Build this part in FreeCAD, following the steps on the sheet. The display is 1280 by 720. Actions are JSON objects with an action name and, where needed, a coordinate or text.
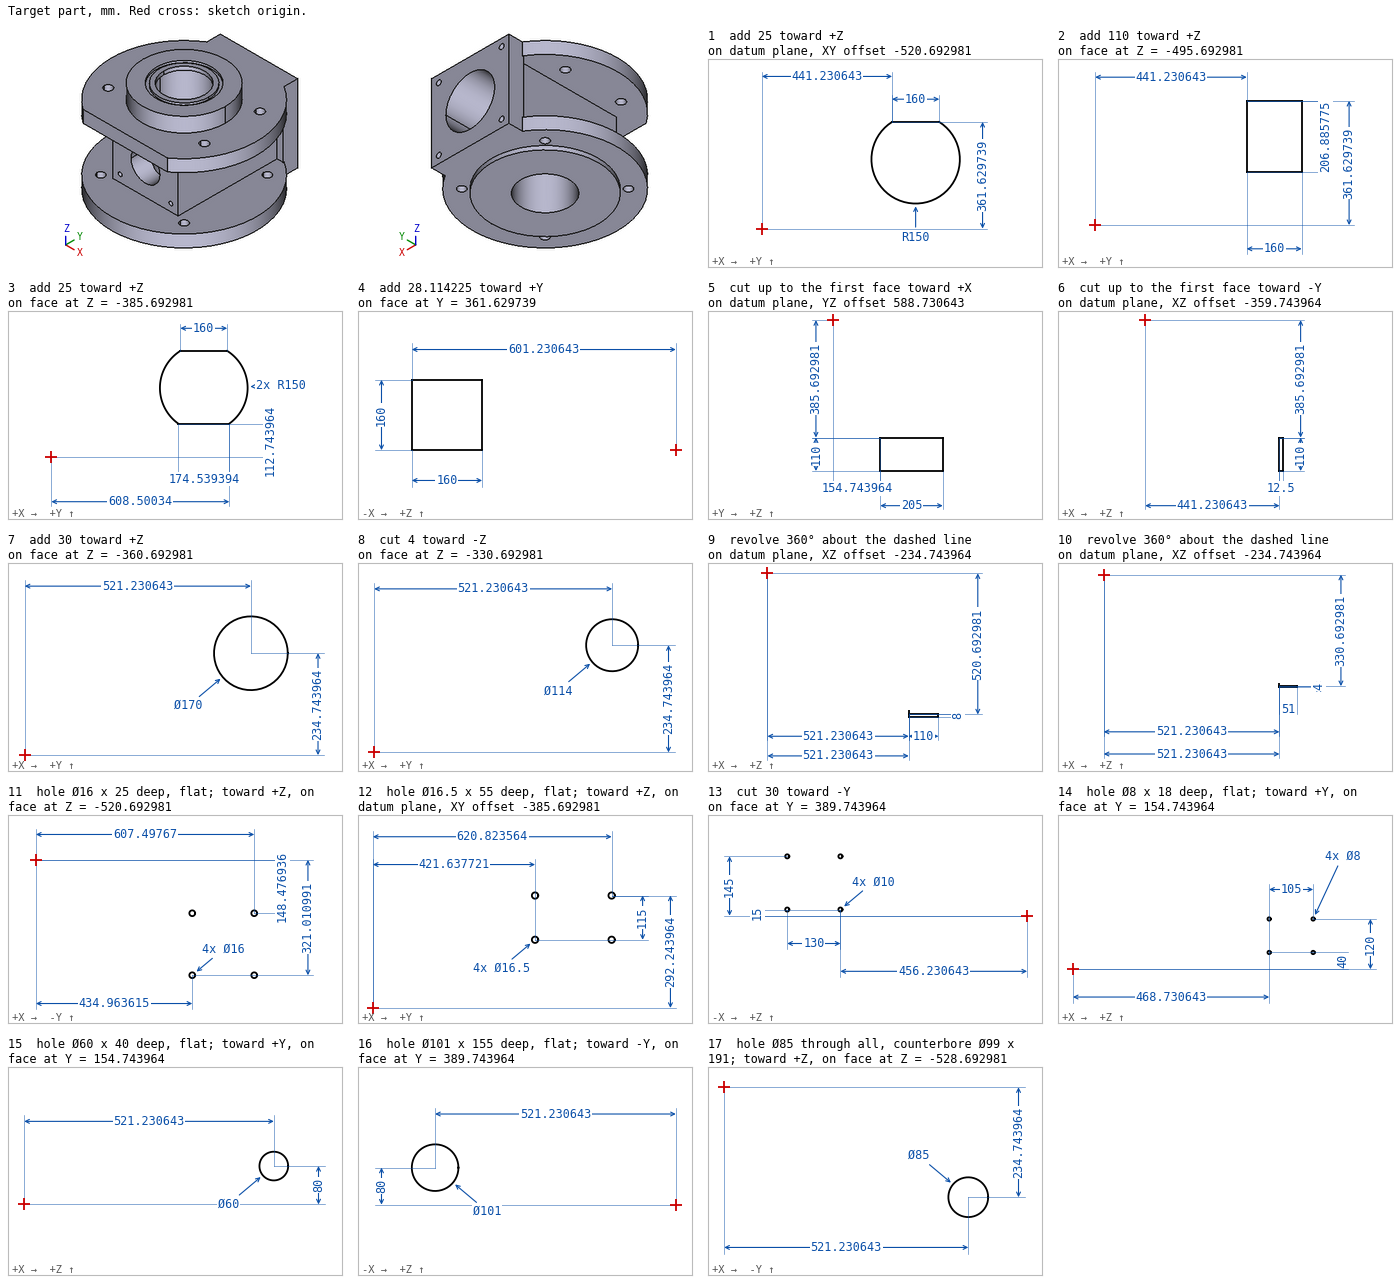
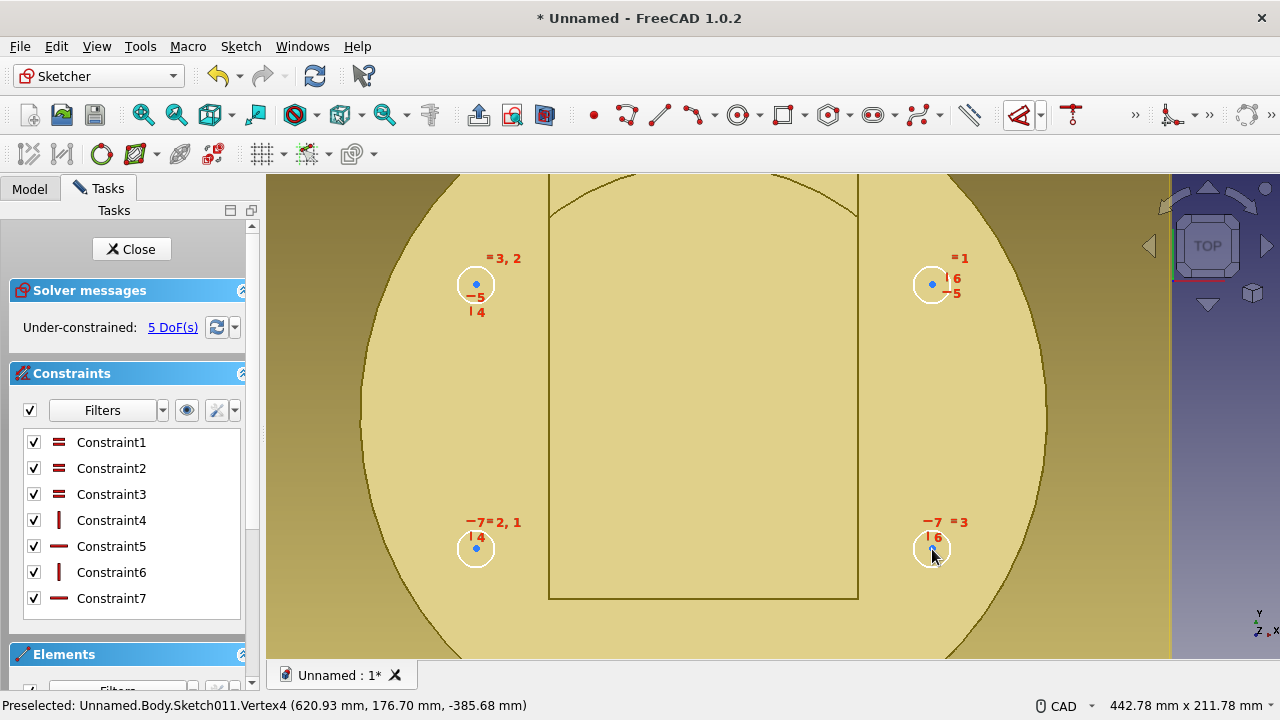
{"action": "left_click", "coordinate": [919, 272]}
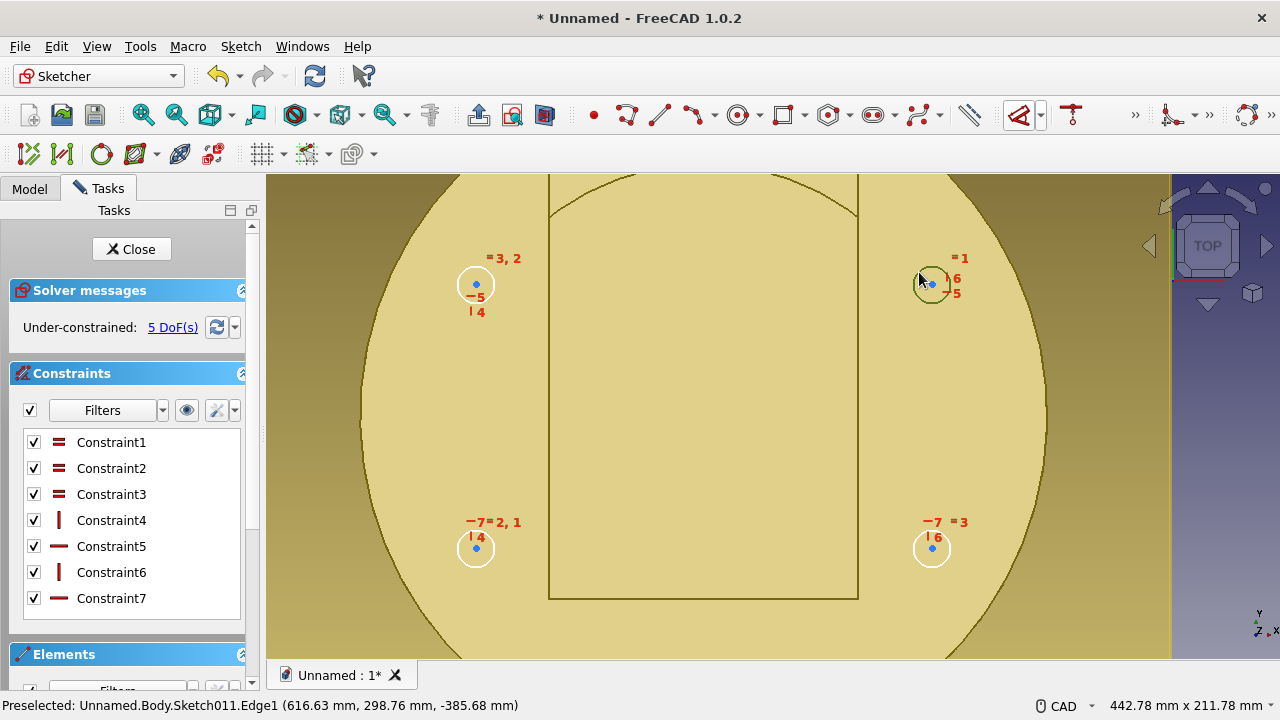
{"action": "left_click", "coordinate": [1040, 116]}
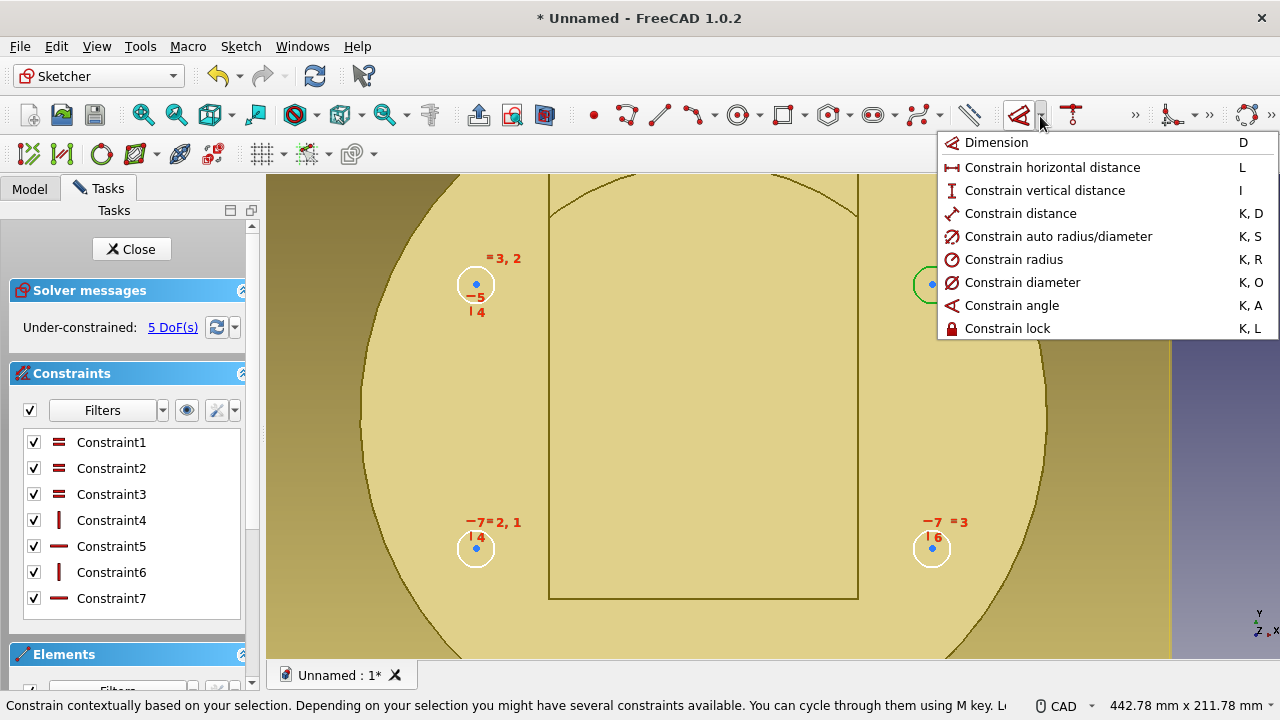
{"action": "left_click", "coordinate": [1108, 282]}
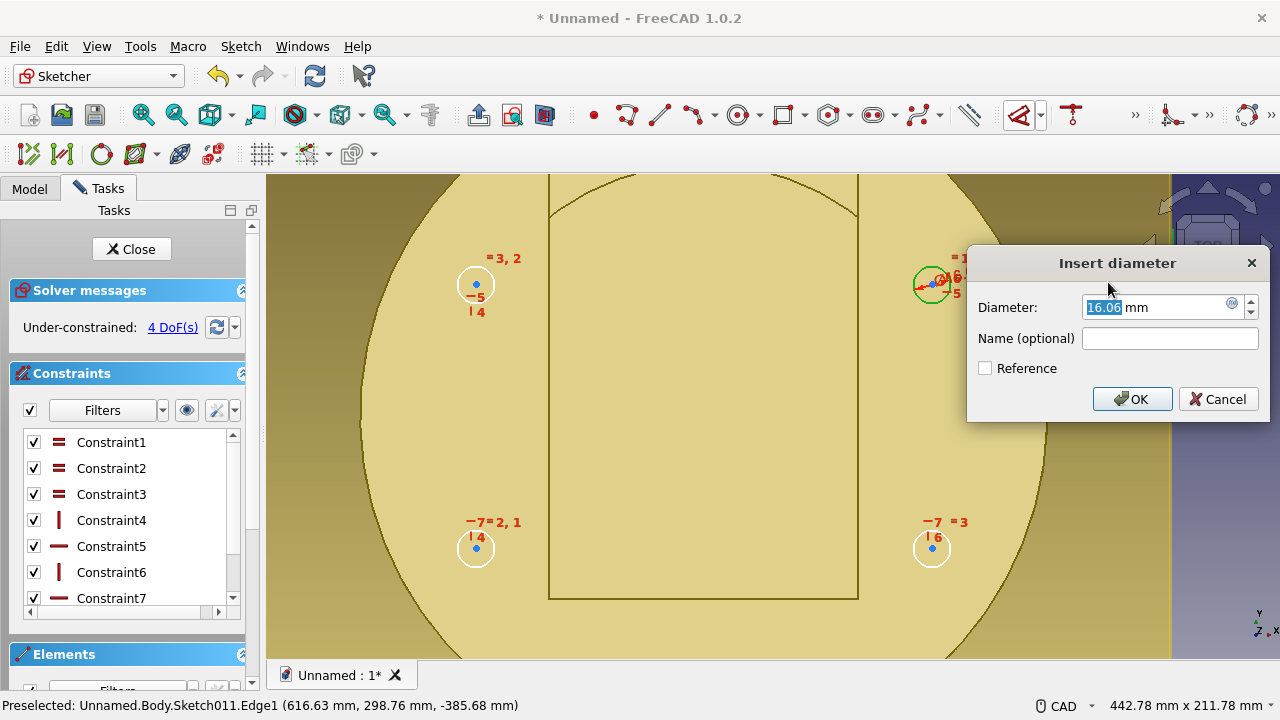
{"action": "type", "text": "16.5"}
{"action": "key", "text": "Return"}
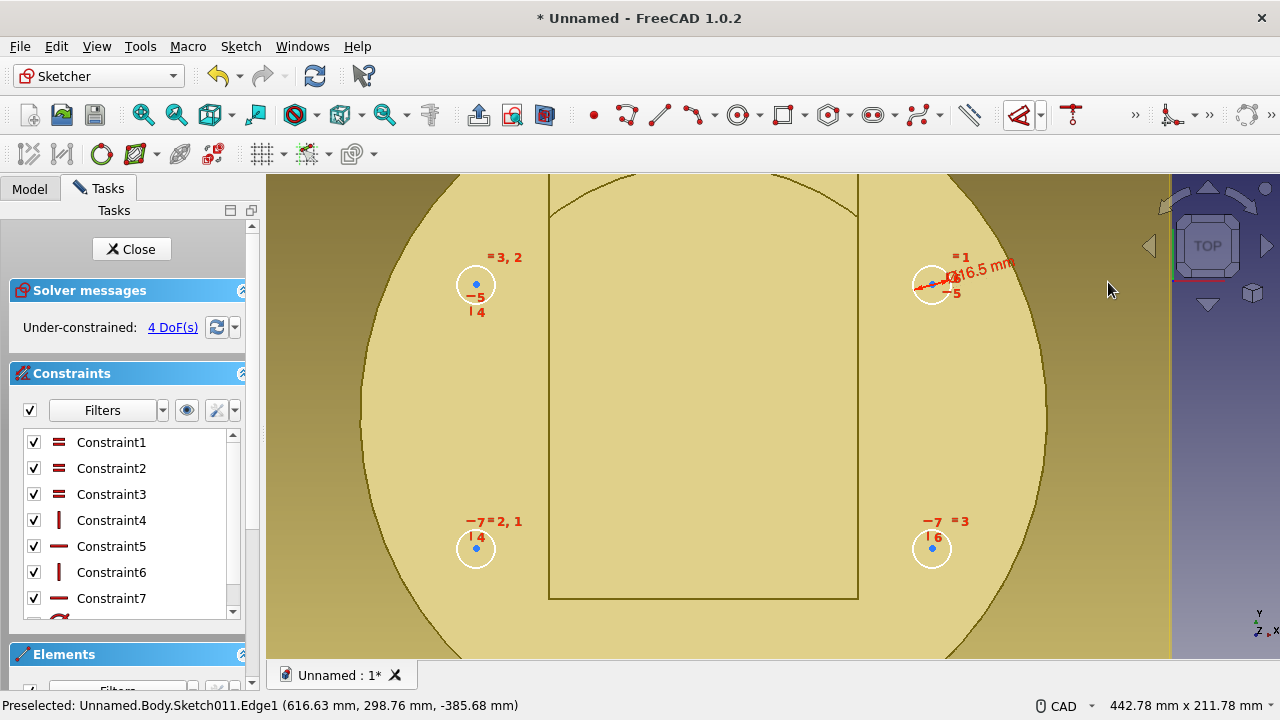
{"action": "left_click", "coordinate": [932, 285]}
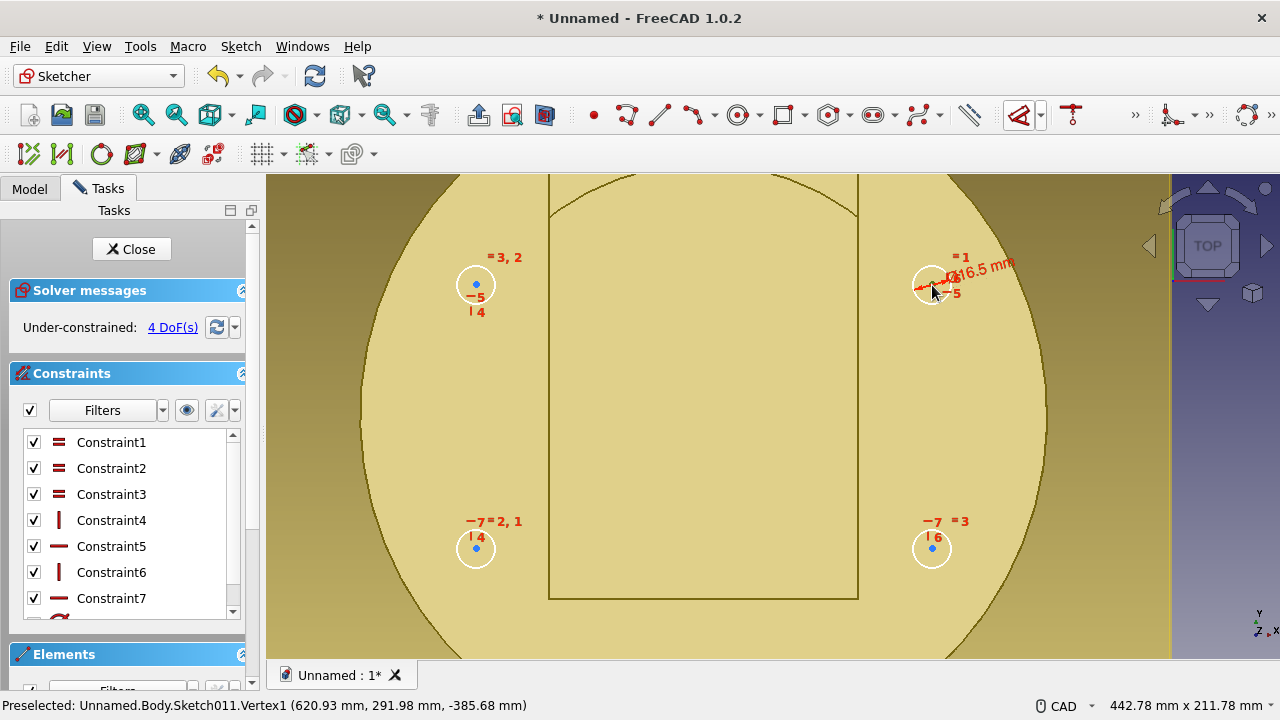
{"action": "left_click", "coordinate": [476, 549]}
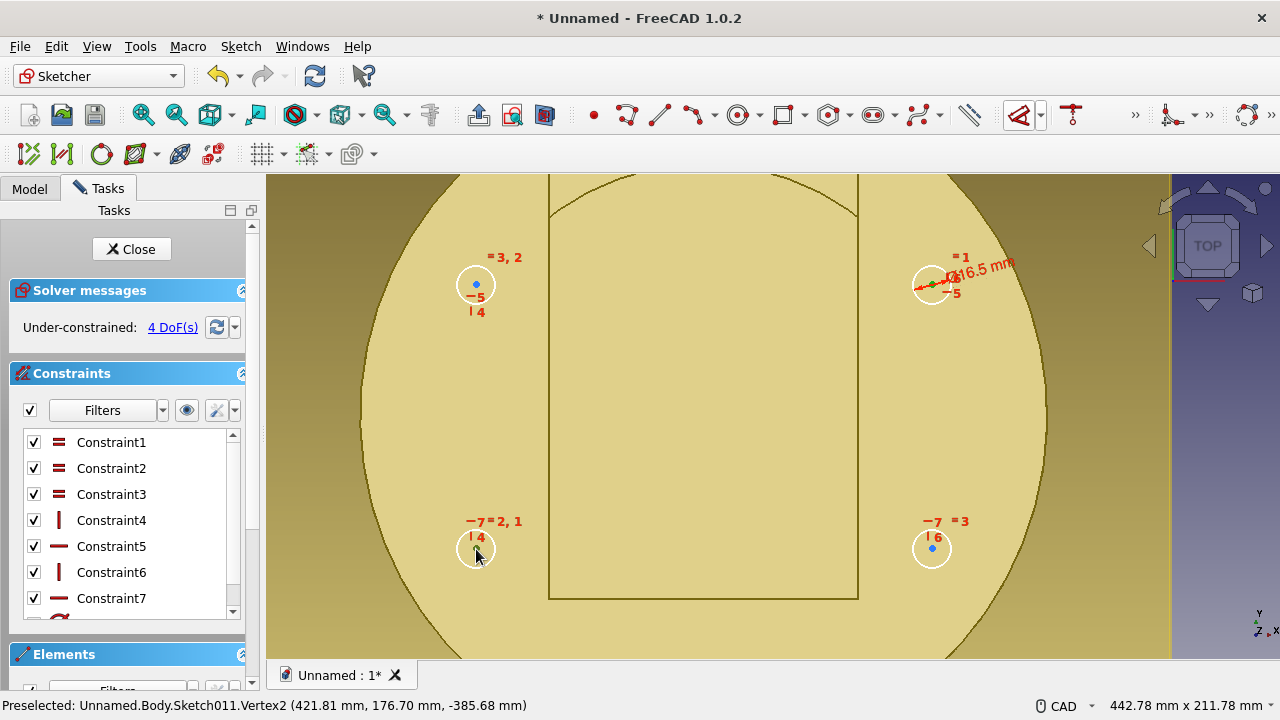
{"action": "left_click", "coordinate": [1040, 116]}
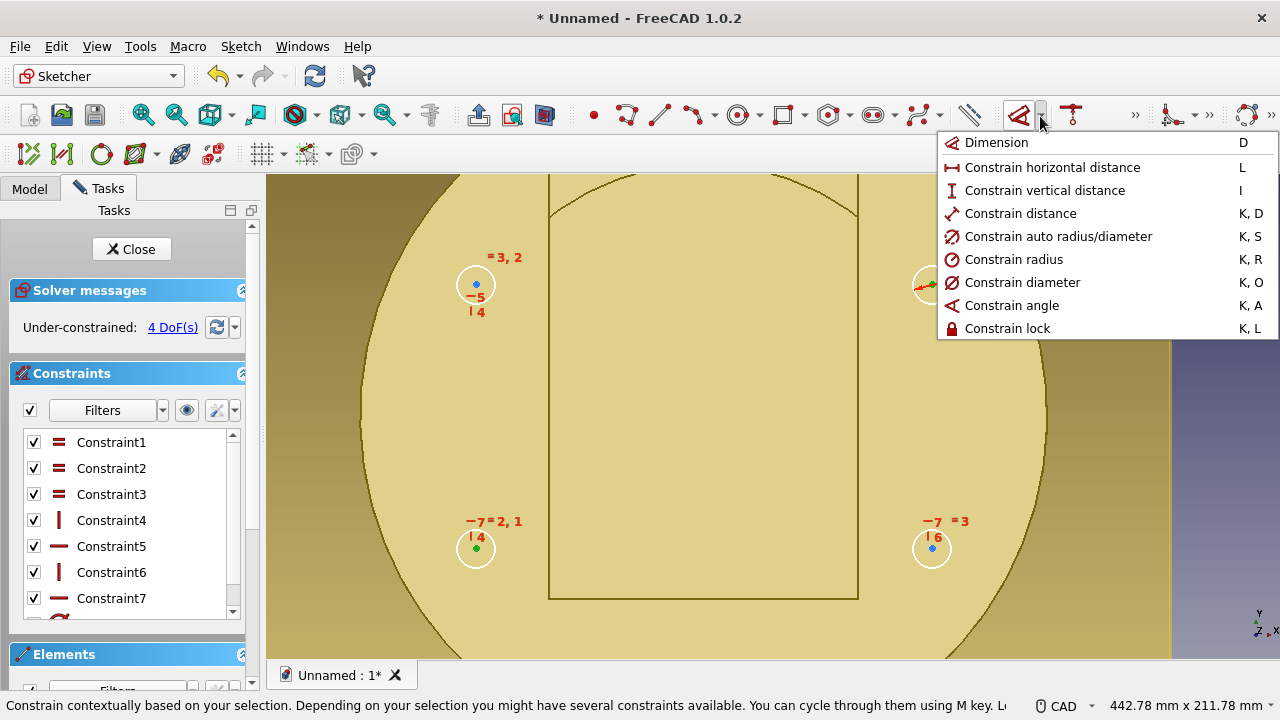
{"action": "left_click", "coordinate": [1108, 190]}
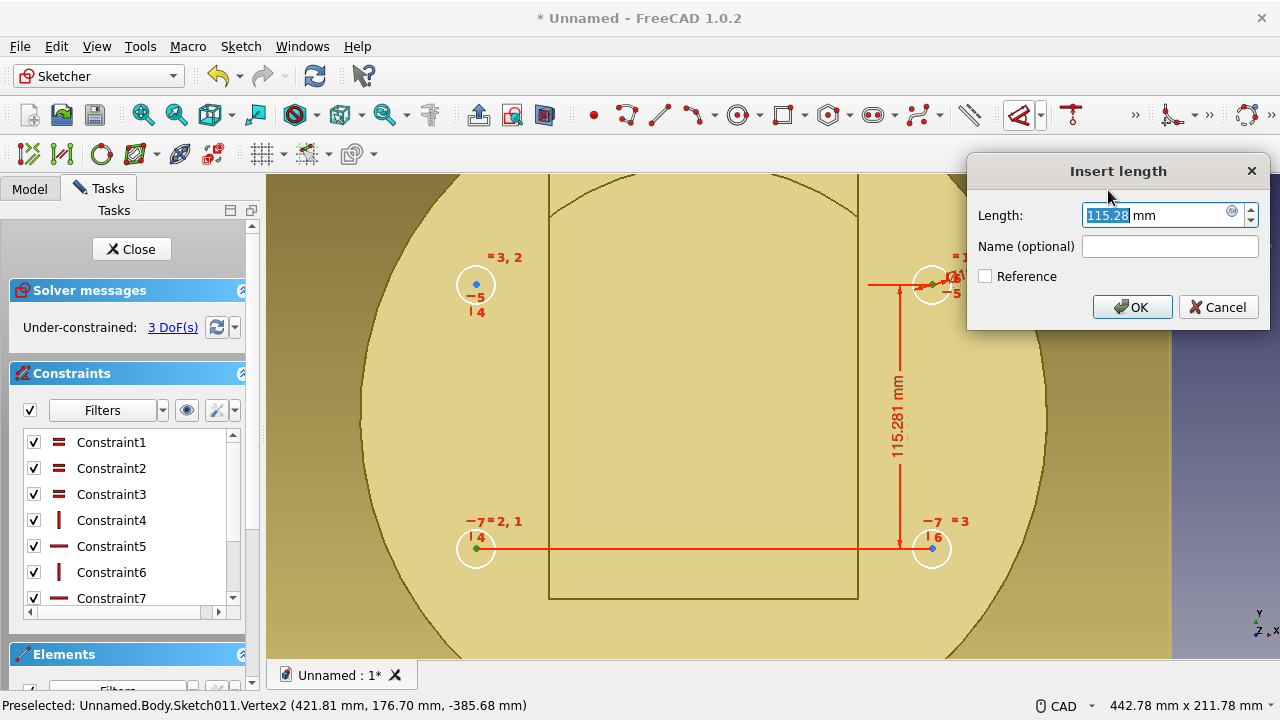
{"action": "type", "text": "115"}
{"action": "key", "text": "Return"}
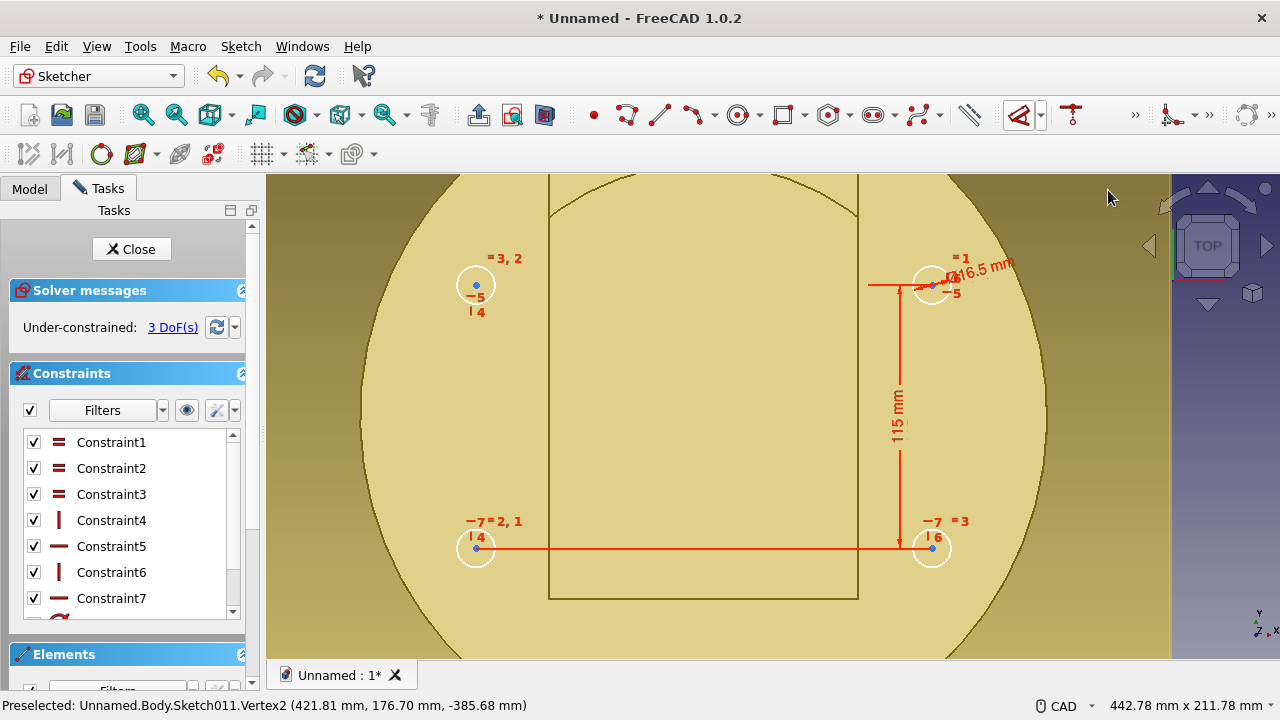
{"action": "left_click", "coordinate": [932, 285]}